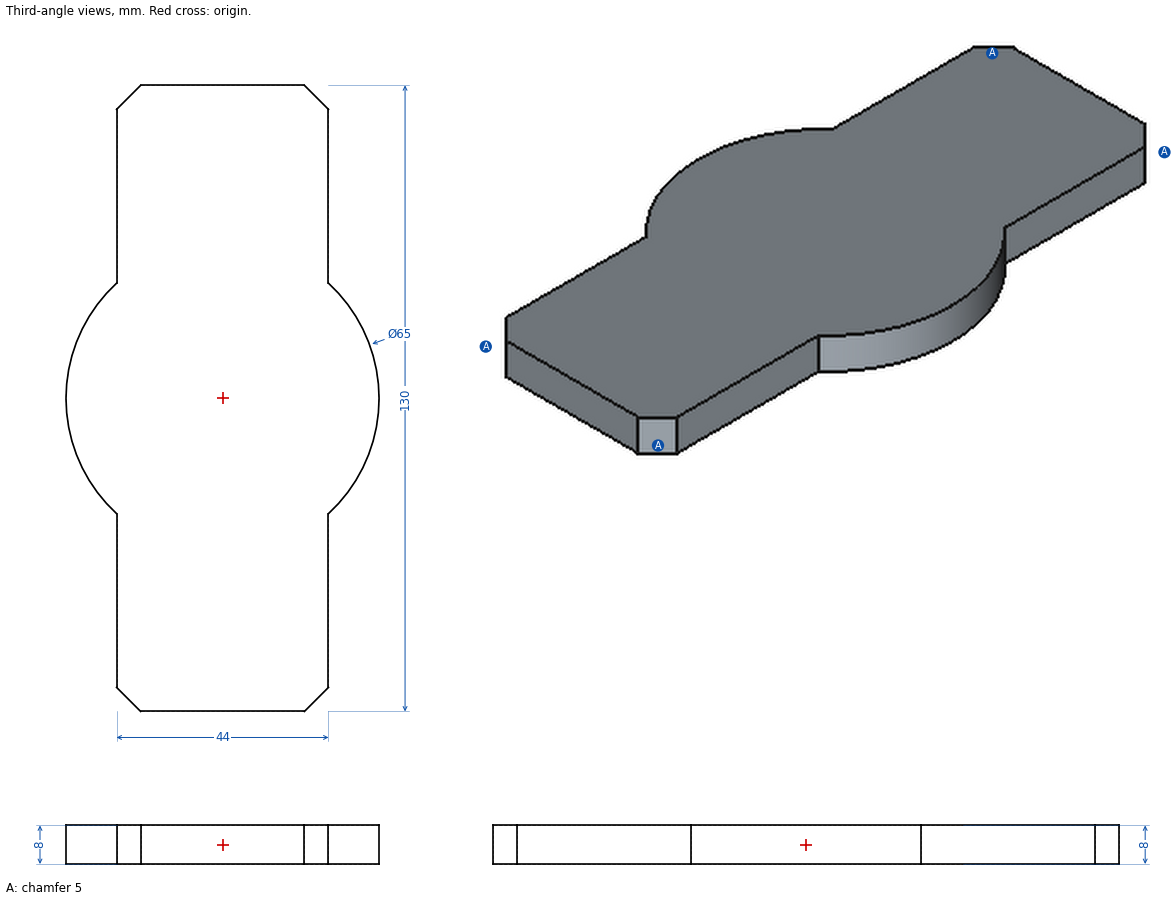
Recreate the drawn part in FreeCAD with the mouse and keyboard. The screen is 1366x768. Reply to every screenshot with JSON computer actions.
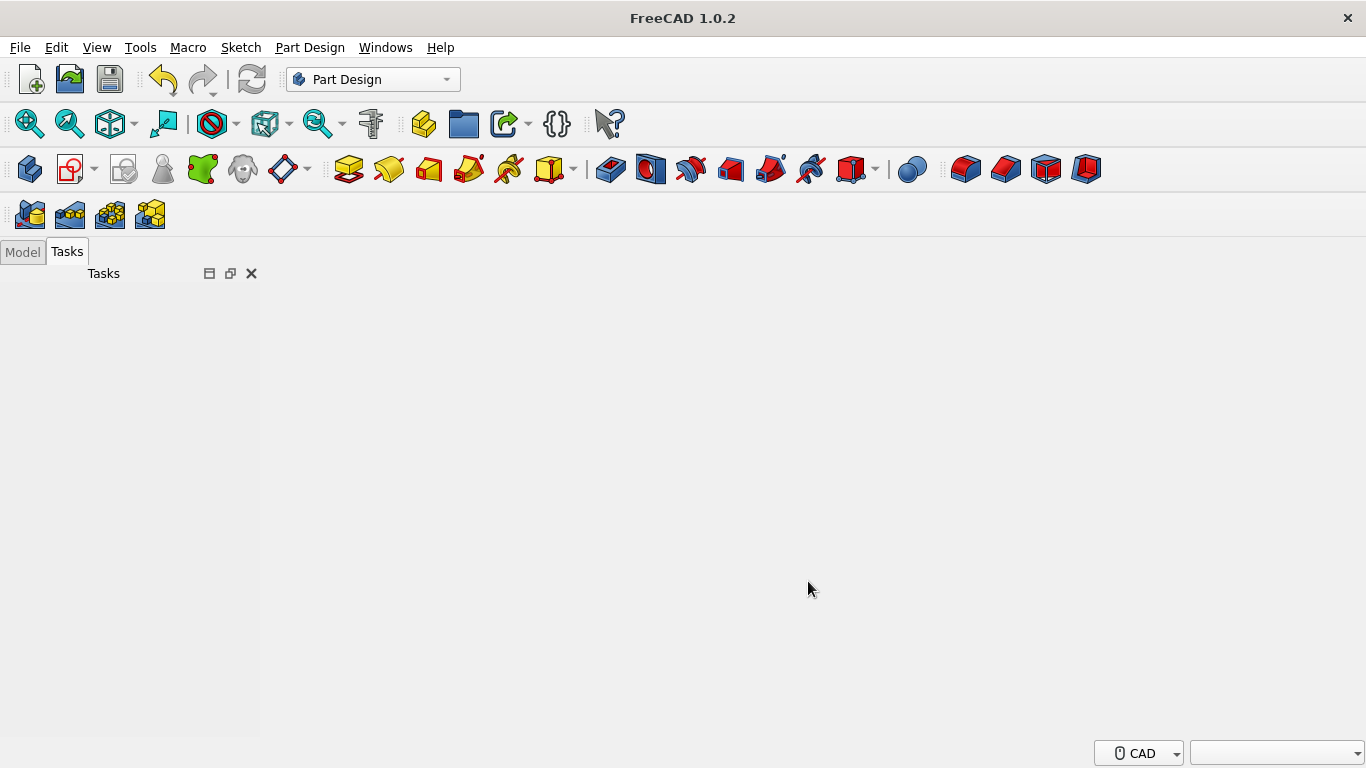
{"action": "left_click", "coordinate": [30, 80]}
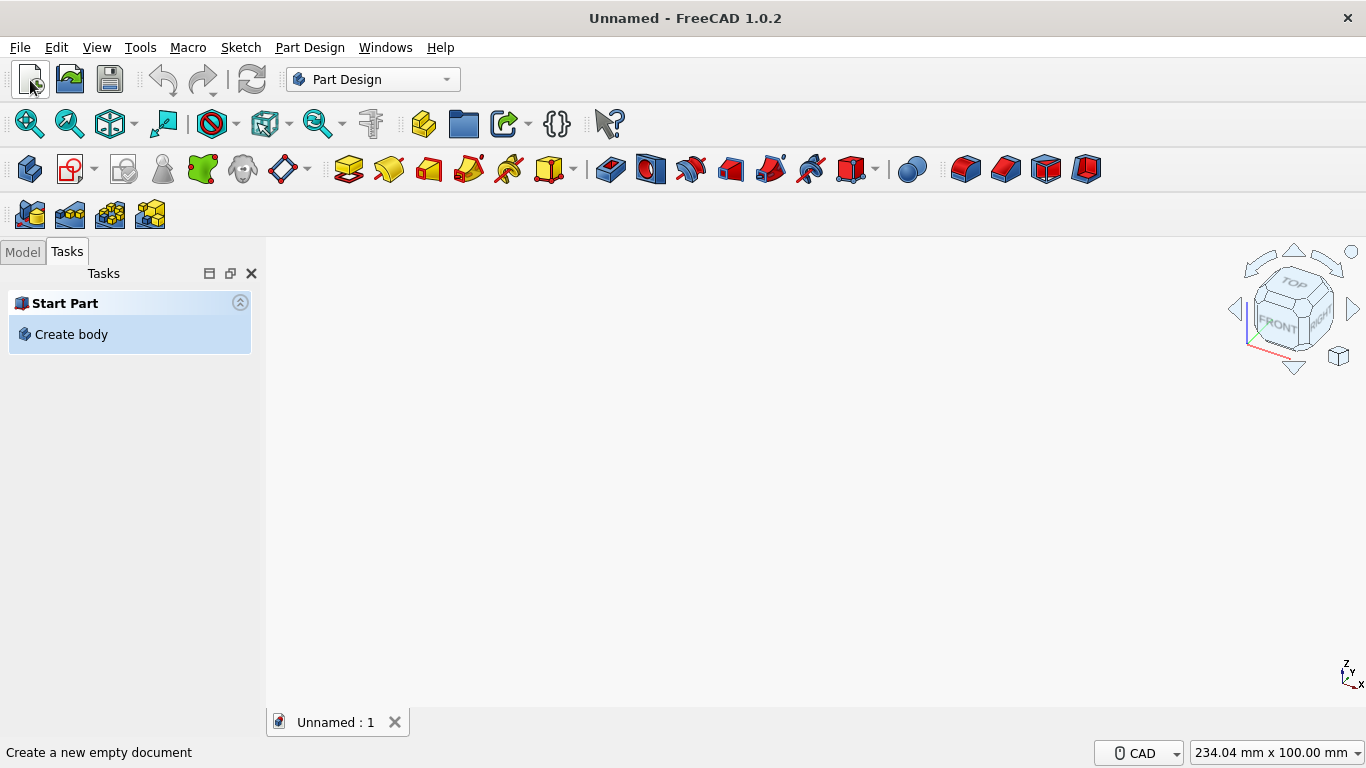
{"action": "left_click", "coordinate": [70, 170]}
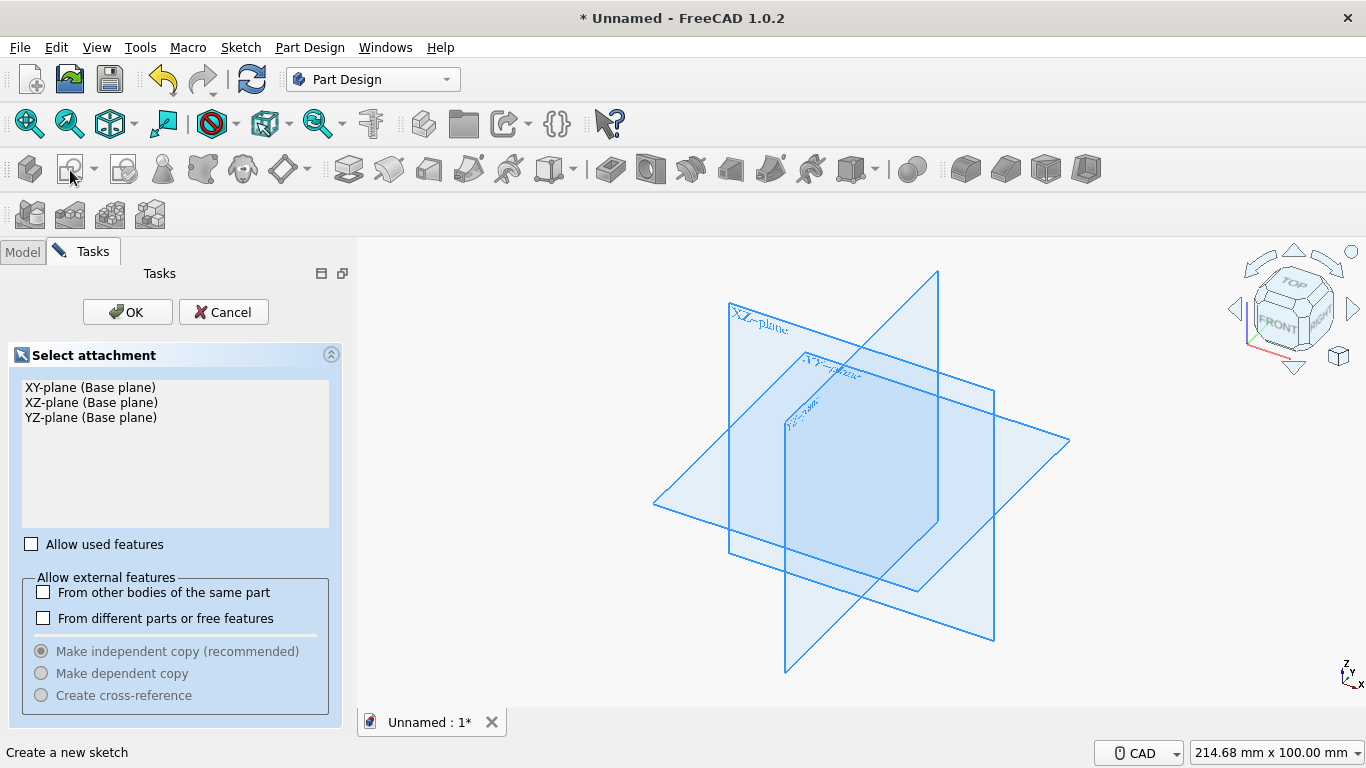
{"action": "left_click", "coordinate": [82, 388]}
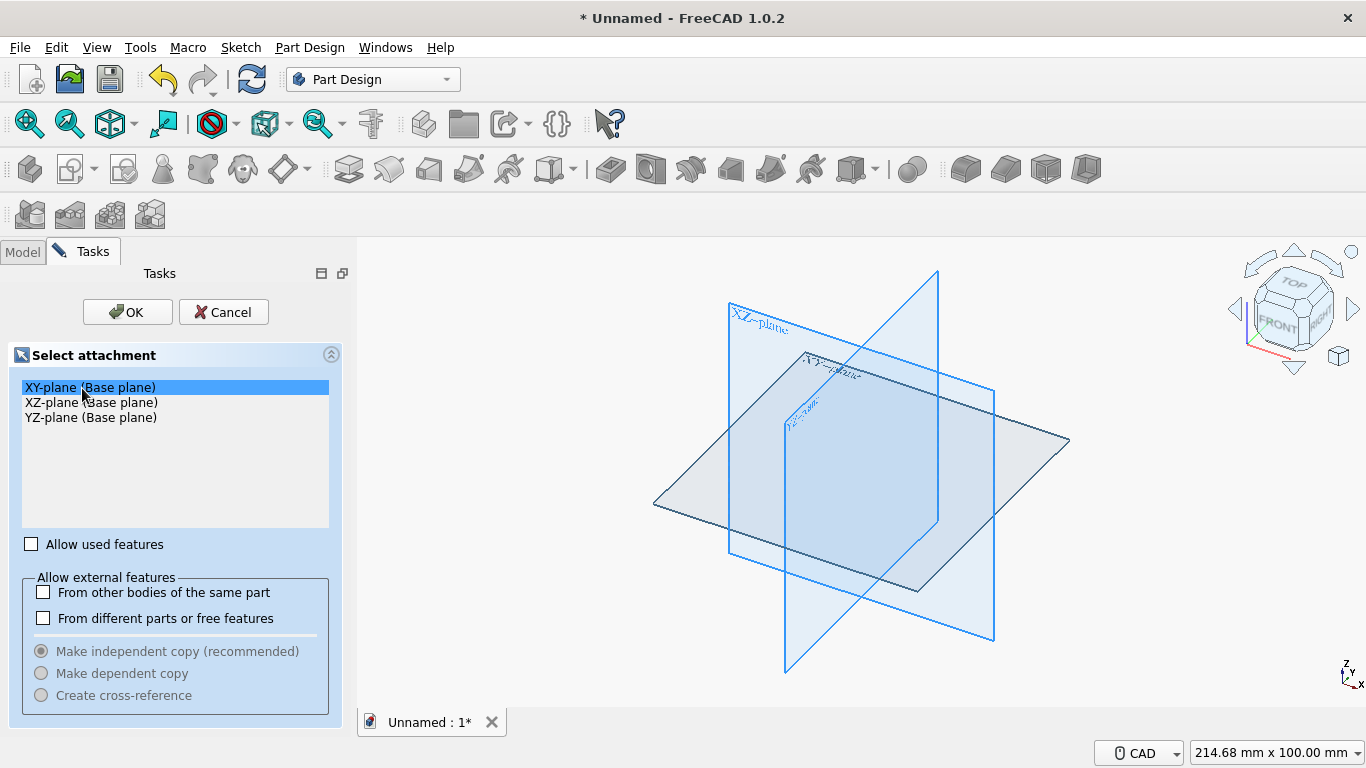
{"action": "left_click", "coordinate": [128, 312]}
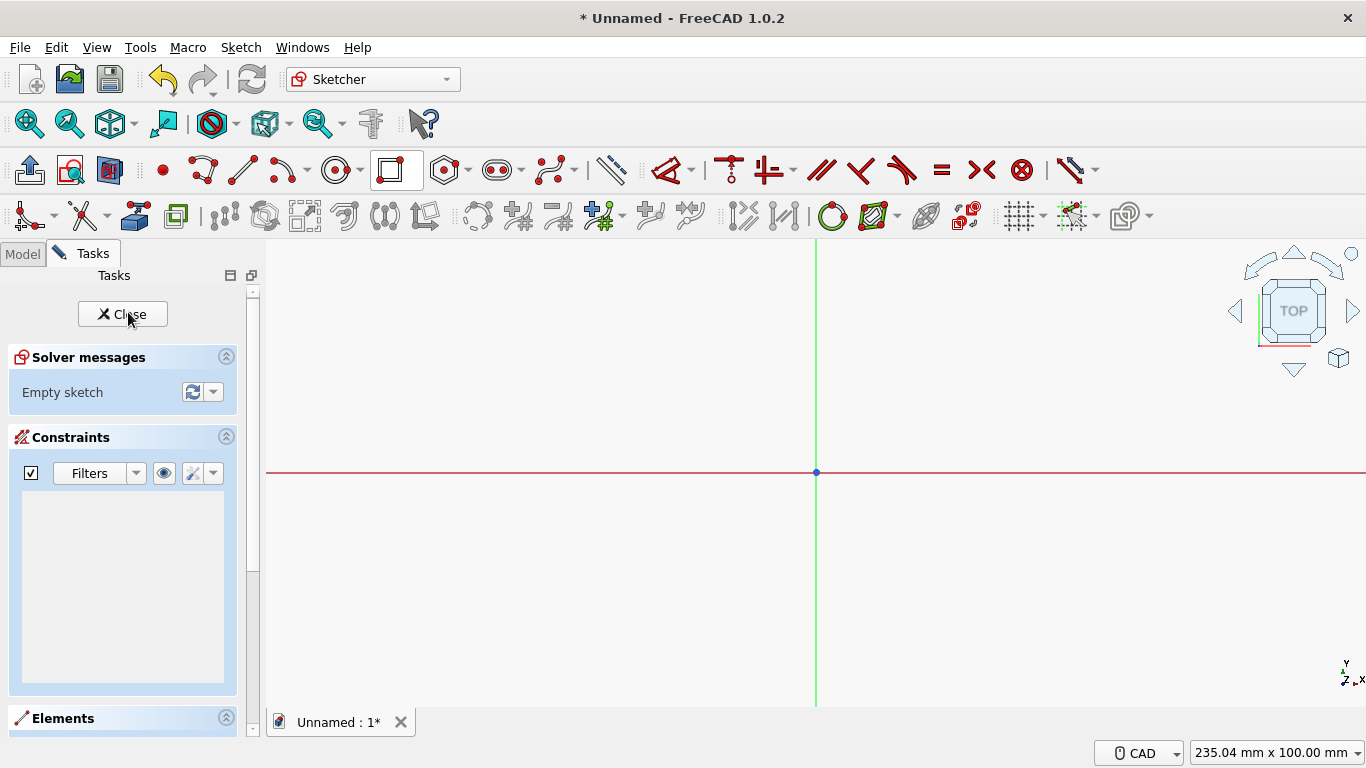
{"action": "left_click", "coordinate": [336, 170]}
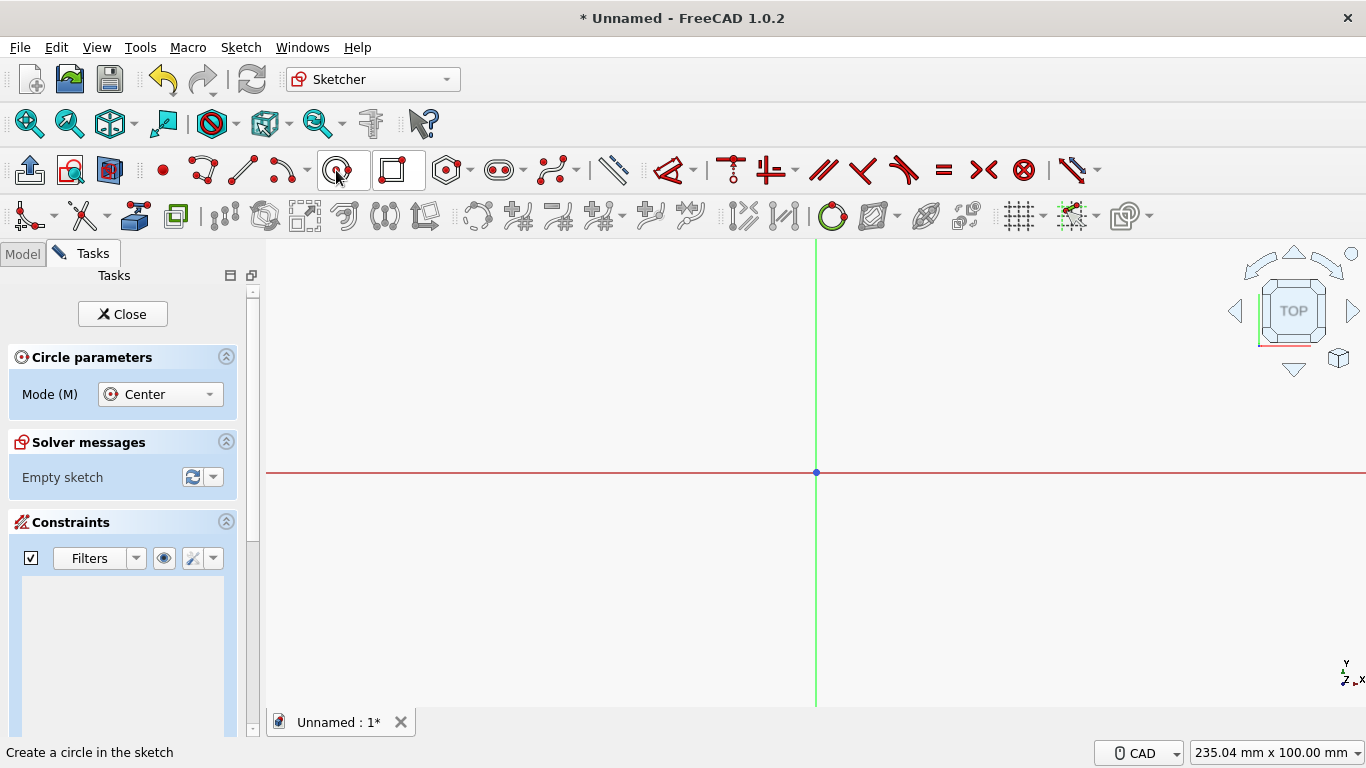
{"action": "left_click", "coordinate": [816, 473]}
{"action": "mouse_move", "coordinate": [924, 365]}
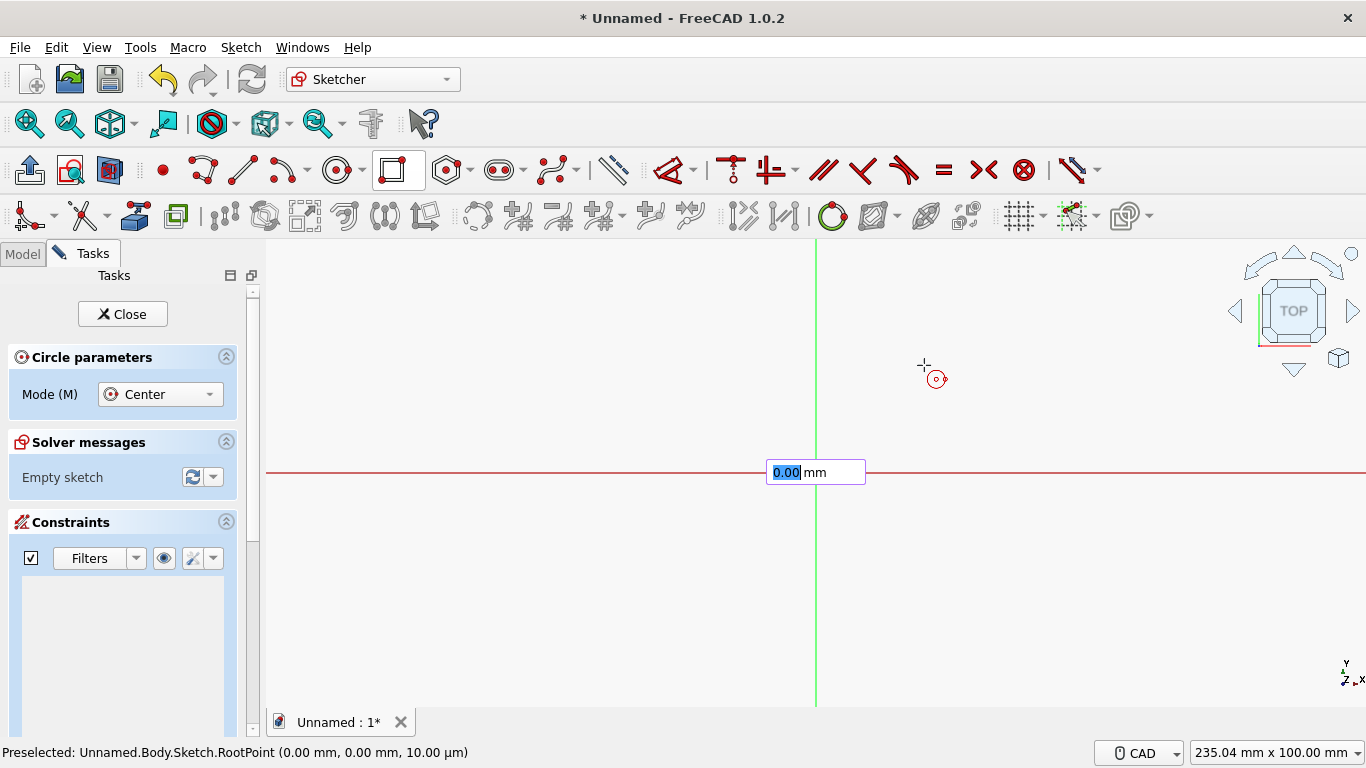
{"action": "type", "text": "65"}
{"action": "key", "text": "Return"}
{"action": "key", "text": "Escape"}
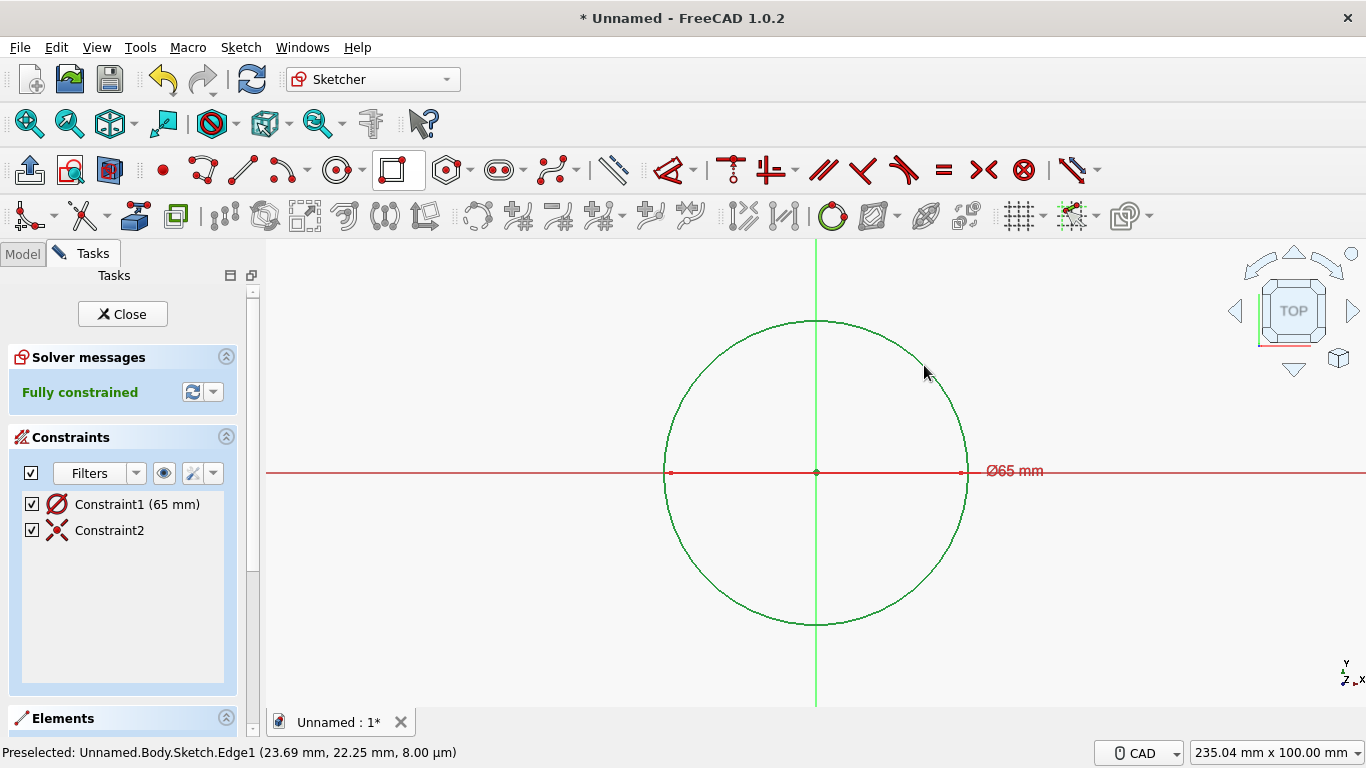
{"action": "left_click", "coordinate": [123, 314]}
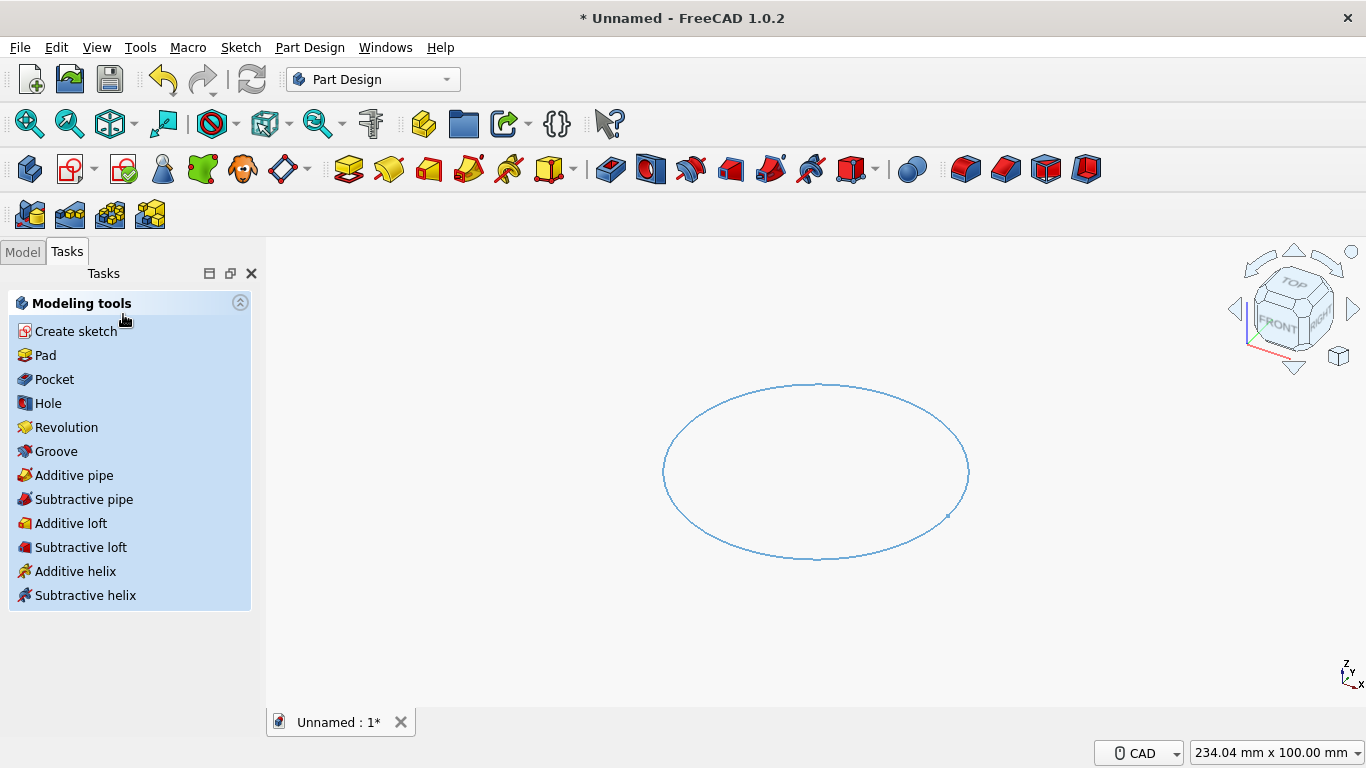
{"action": "left_click", "coordinate": [350, 170]}